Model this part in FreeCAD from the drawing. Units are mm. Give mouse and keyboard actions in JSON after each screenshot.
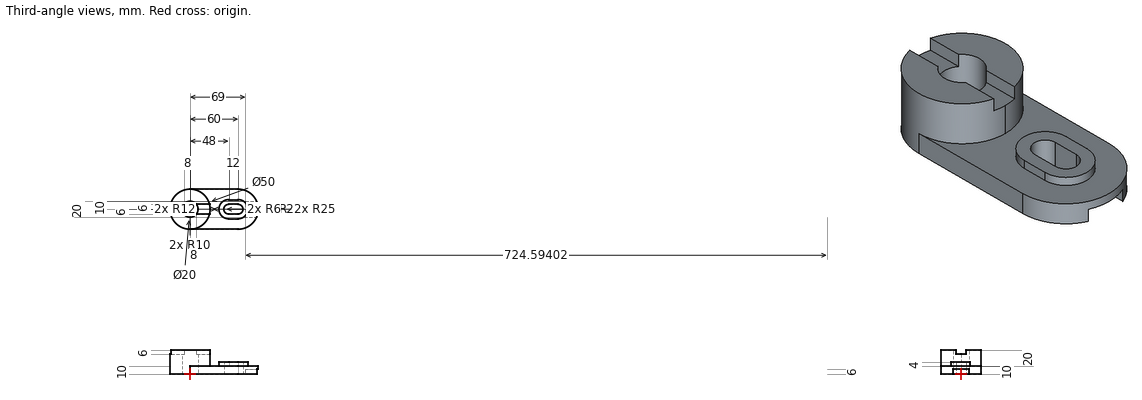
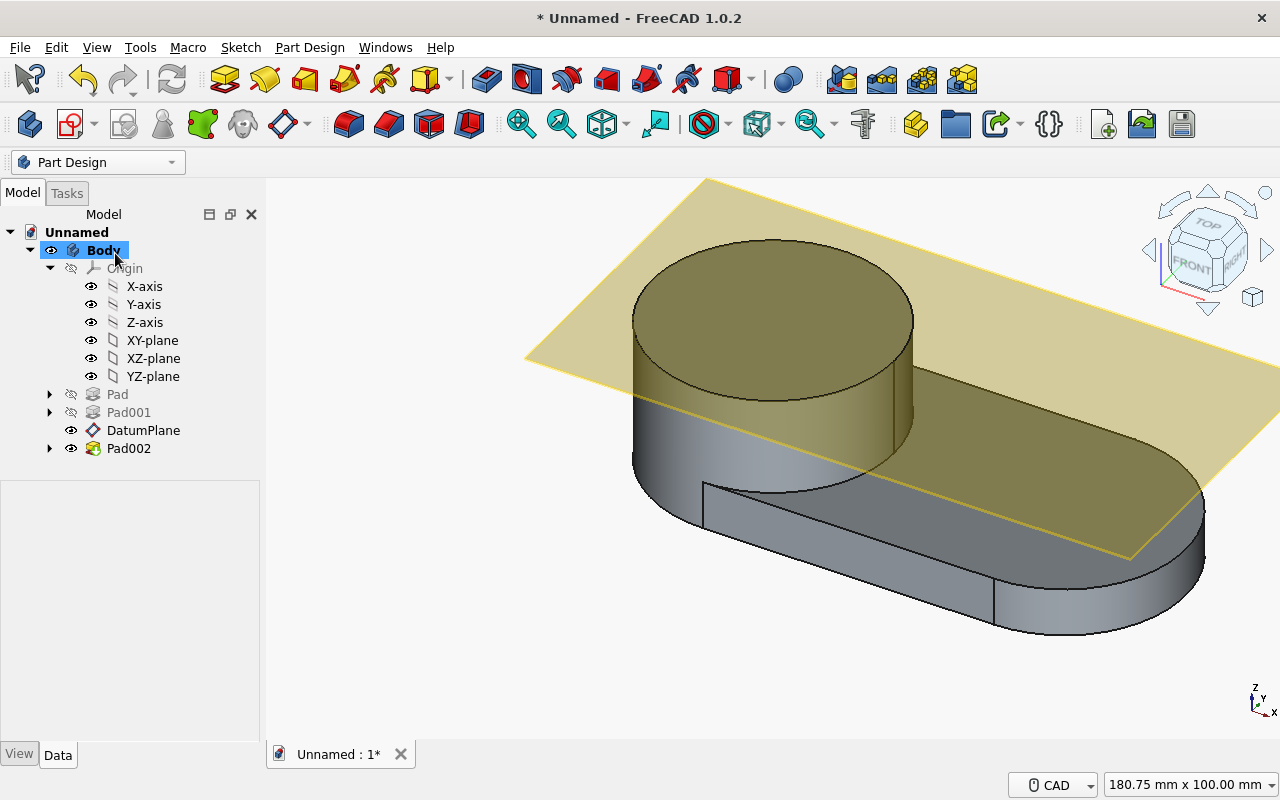
{"action": "left_click", "coordinate": [116, 430]}
{"action": "key", "text": "space"}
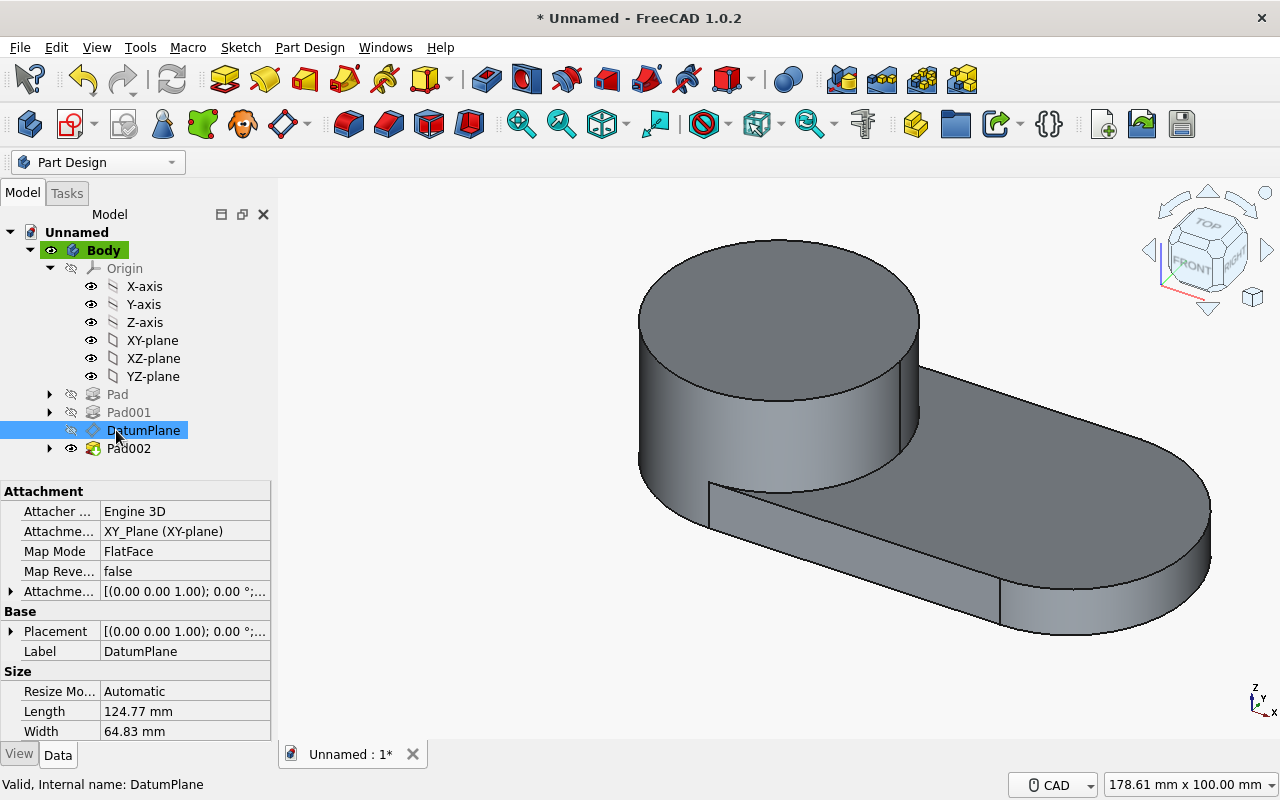
{"action": "left_click", "coordinate": [779, 320]}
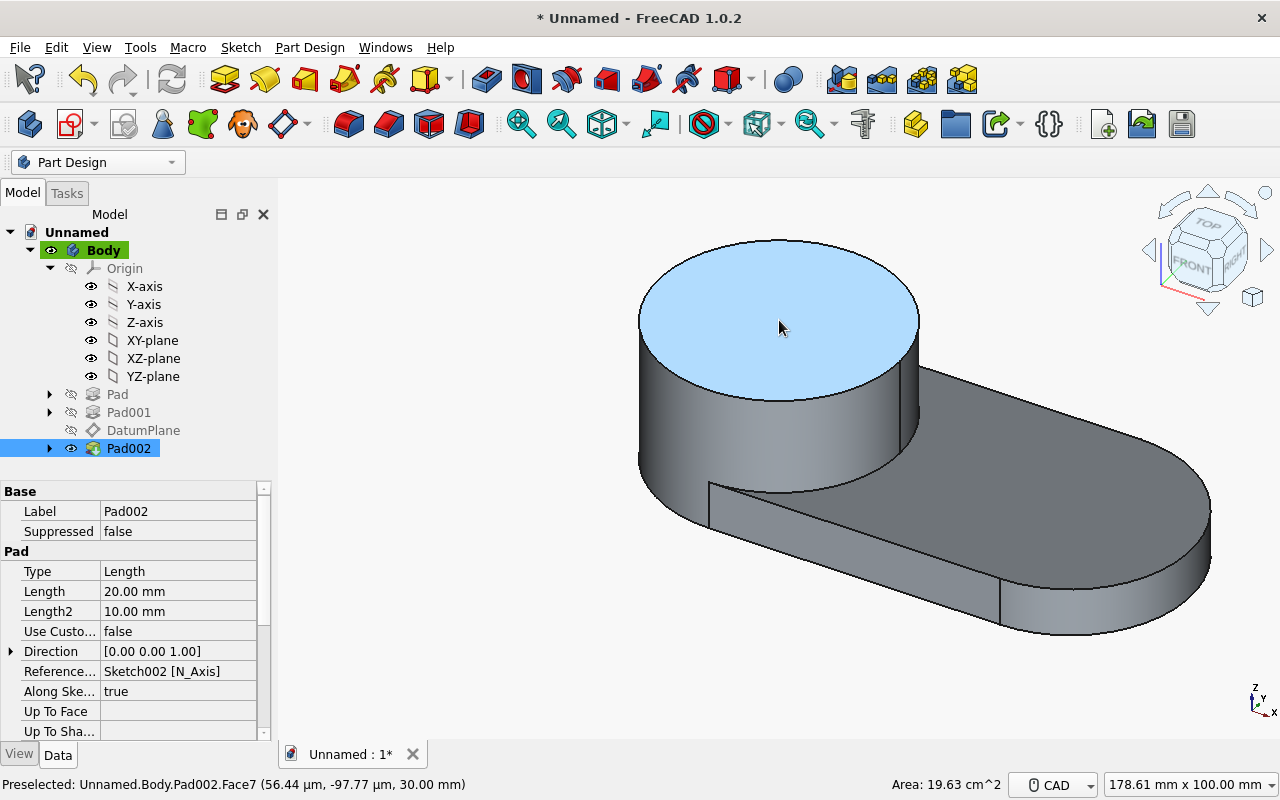
{"action": "left_click", "coordinate": [70, 124]}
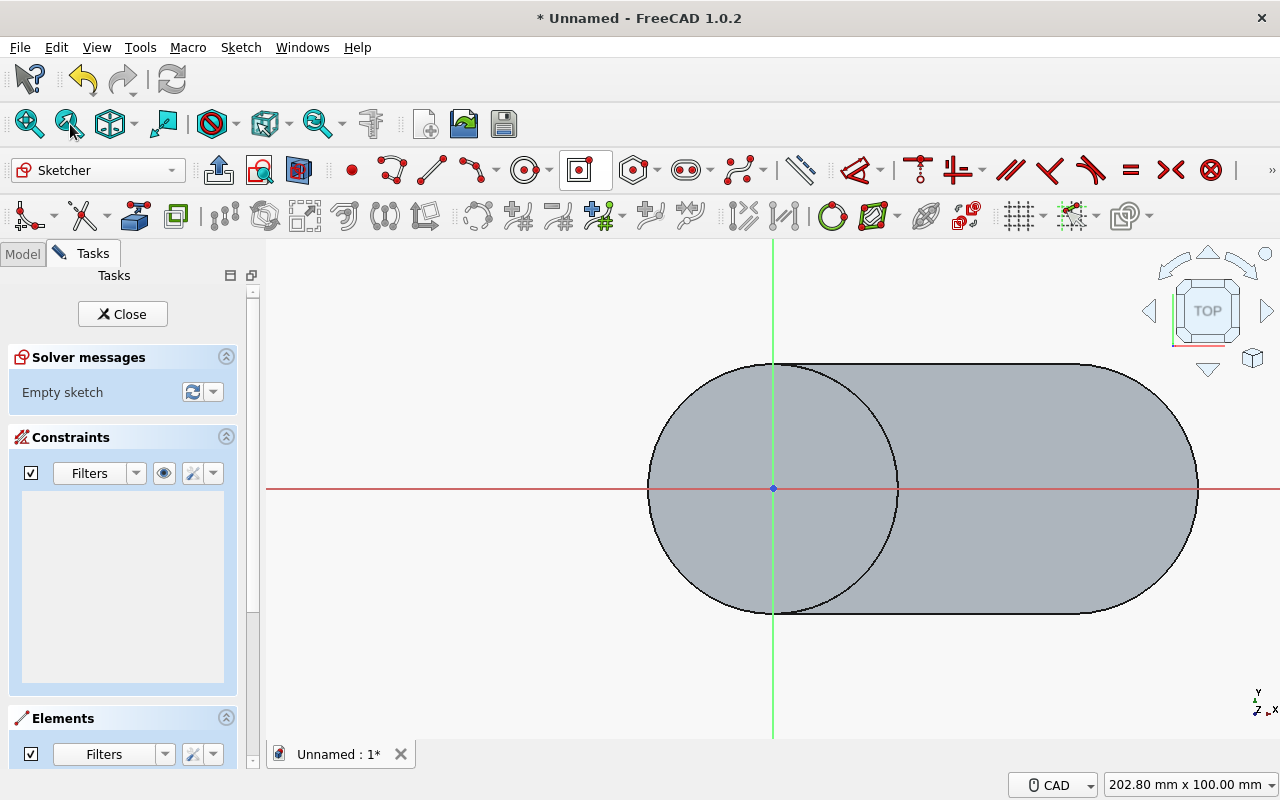
{"action": "scroll", "coordinate": [829, 489], "scroll_direction": "up", "scroll_amount": 4}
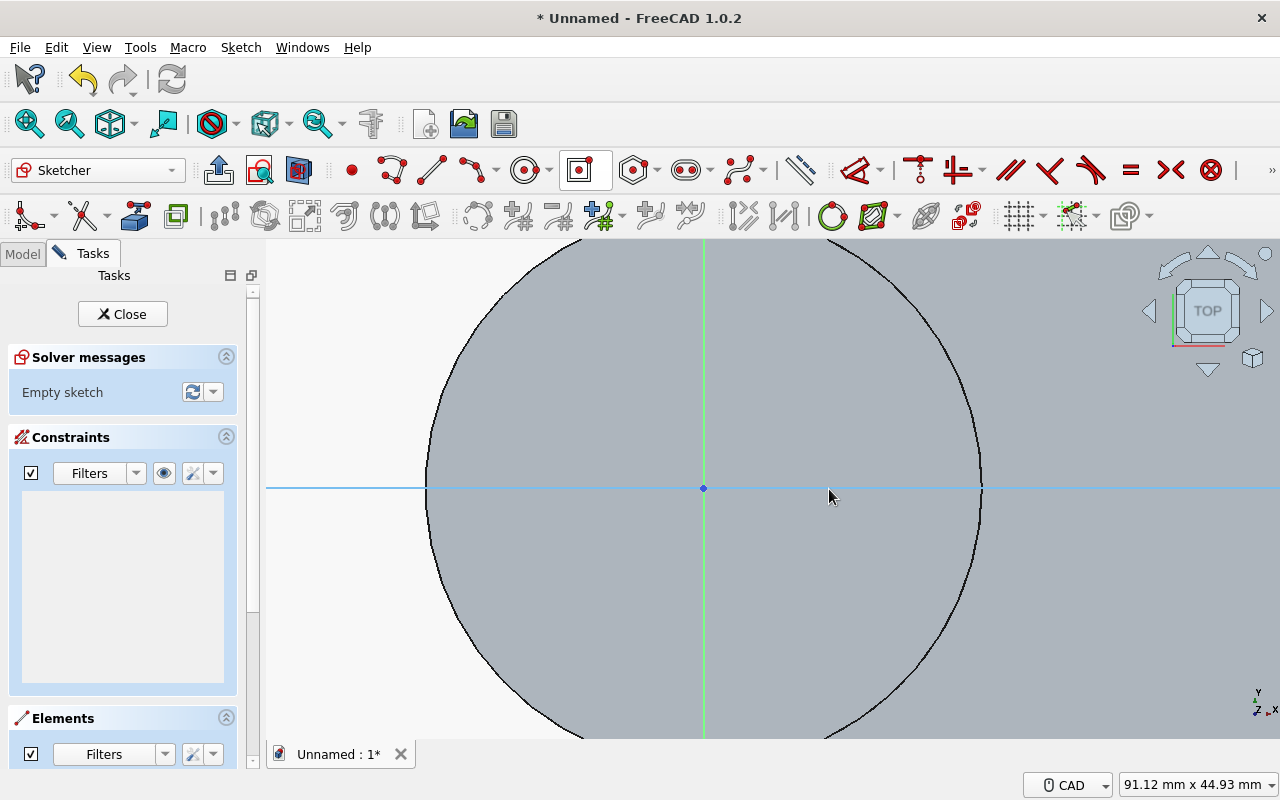
{"action": "left_click", "coordinate": [432, 170]}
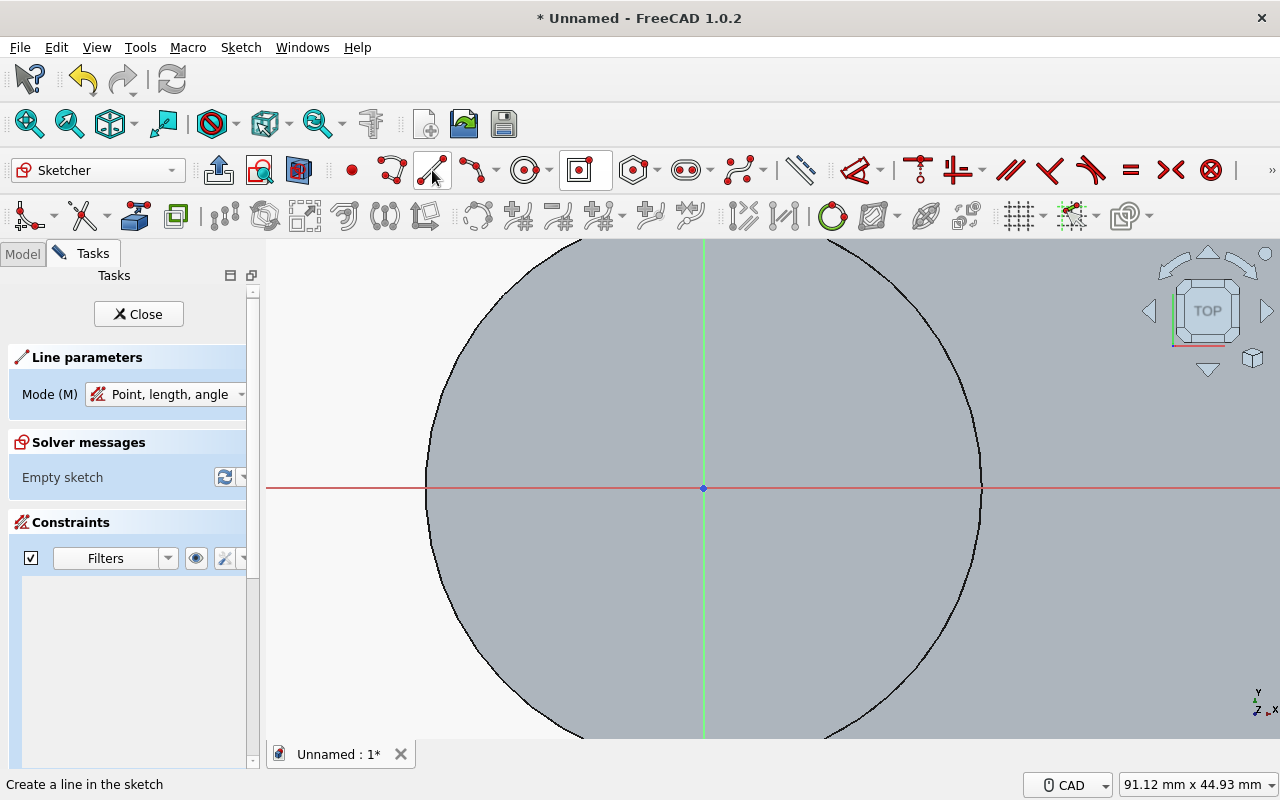
{"action": "left_click", "coordinate": [974, 422]}
{"action": "left_click", "coordinate": [793, 422]}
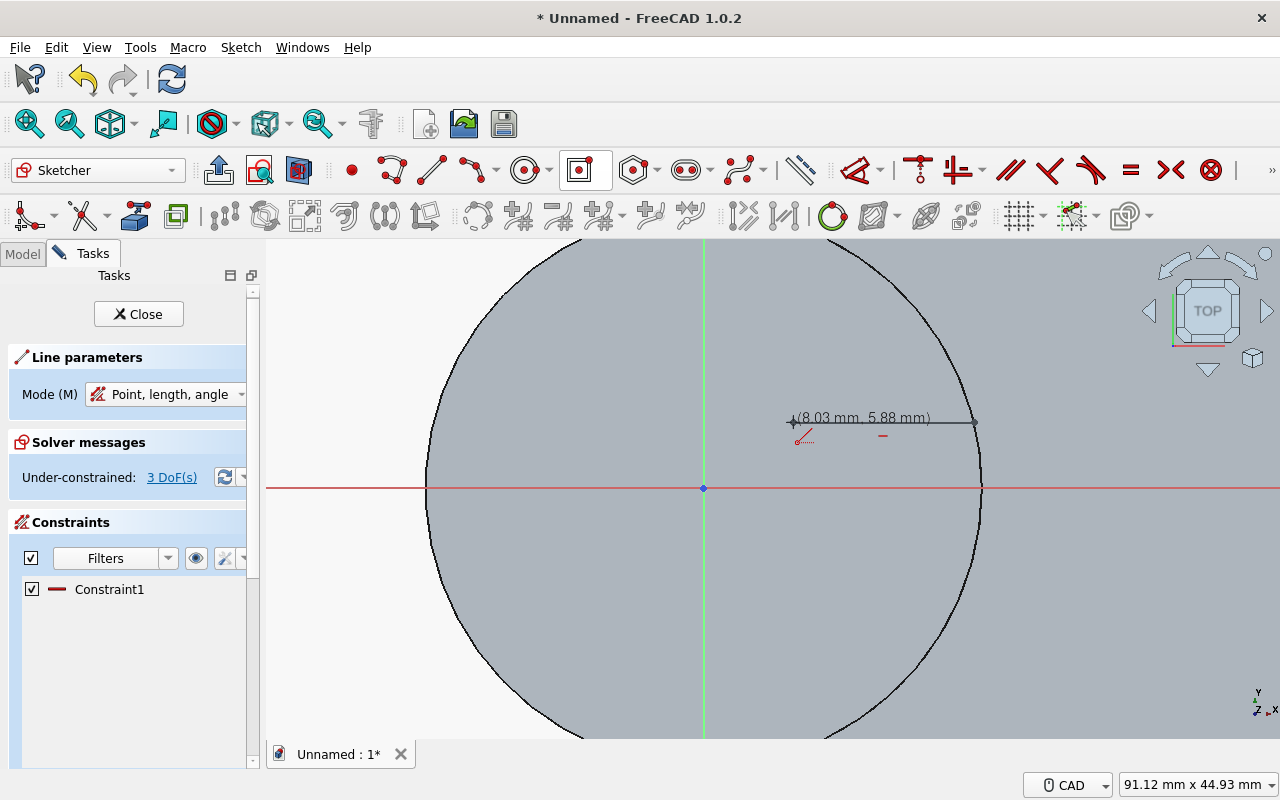
{"action": "left_click", "coordinate": [615, 422]}
{"action": "left_click", "coordinate": [434, 422]}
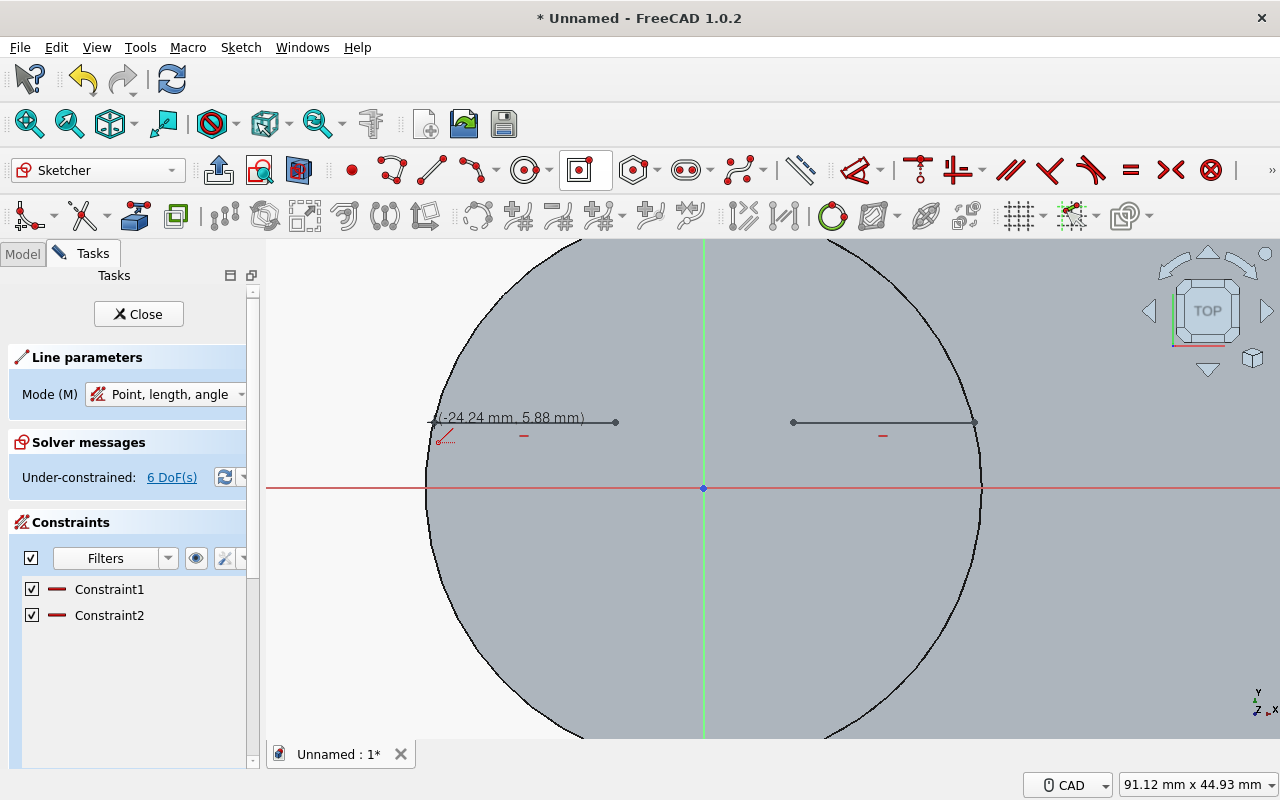
{"action": "left_click", "coordinate": [434, 555]}
{"action": "left_click", "coordinate": [615, 555]}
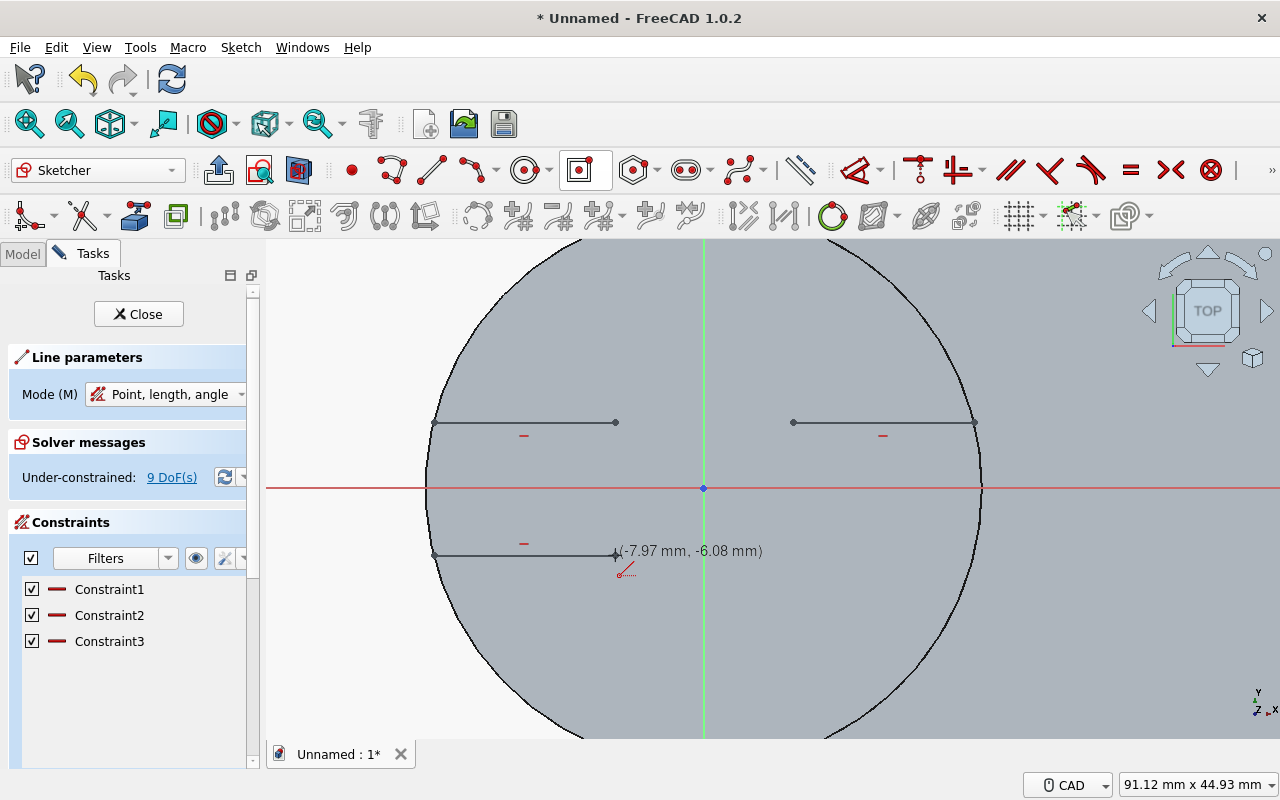
{"action": "left_click", "coordinate": [793, 555]}
{"action": "left_click", "coordinate": [974, 555]}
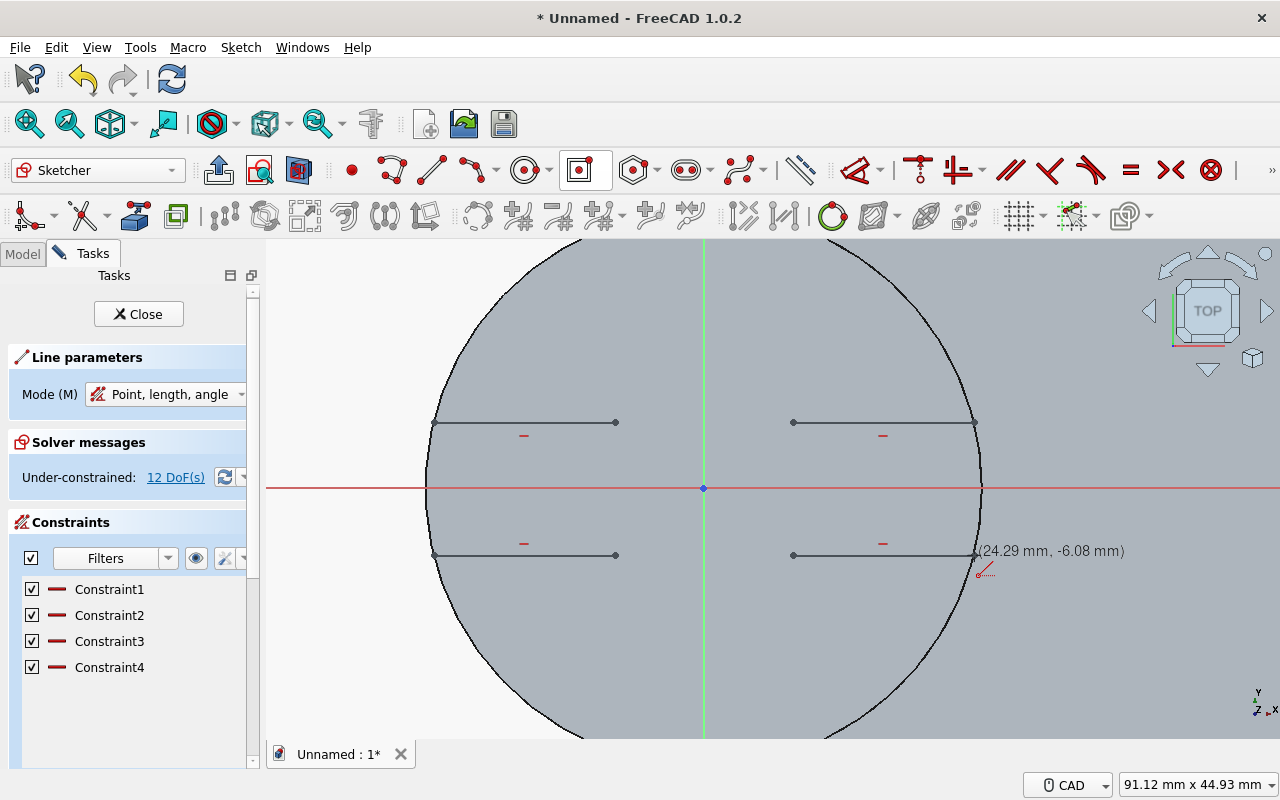
{"action": "left_click", "coordinate": [472, 170]}